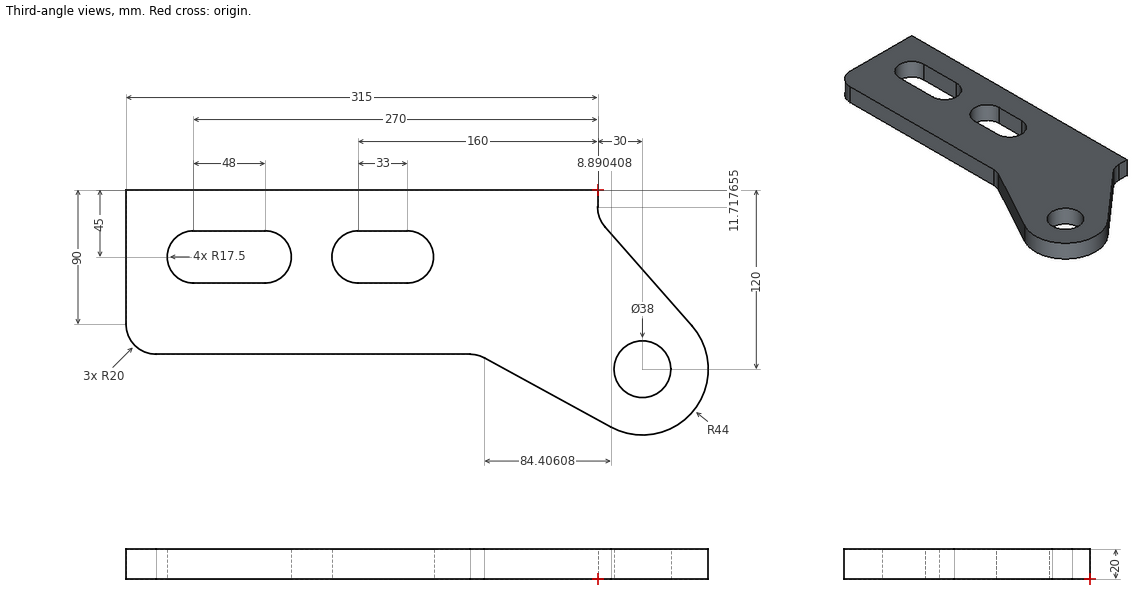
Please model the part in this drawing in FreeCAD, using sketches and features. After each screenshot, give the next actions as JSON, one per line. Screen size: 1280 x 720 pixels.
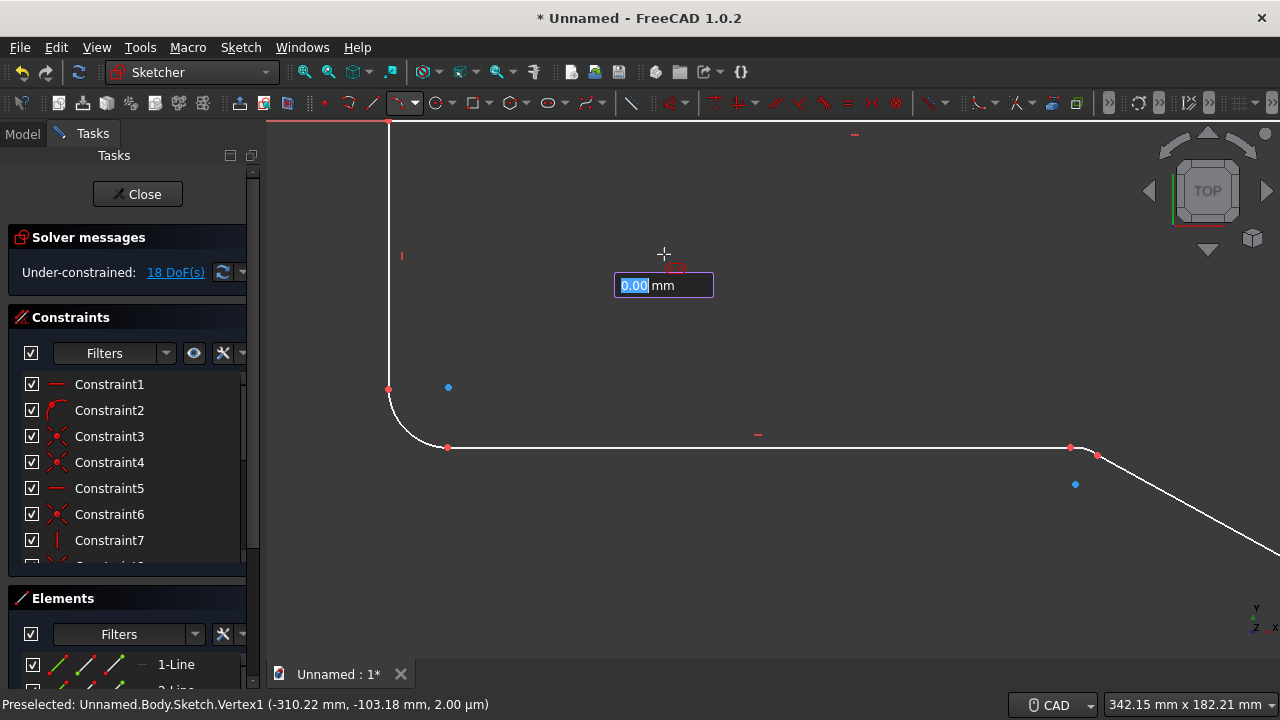
{"action": "left_click", "coordinate": [593, 202]}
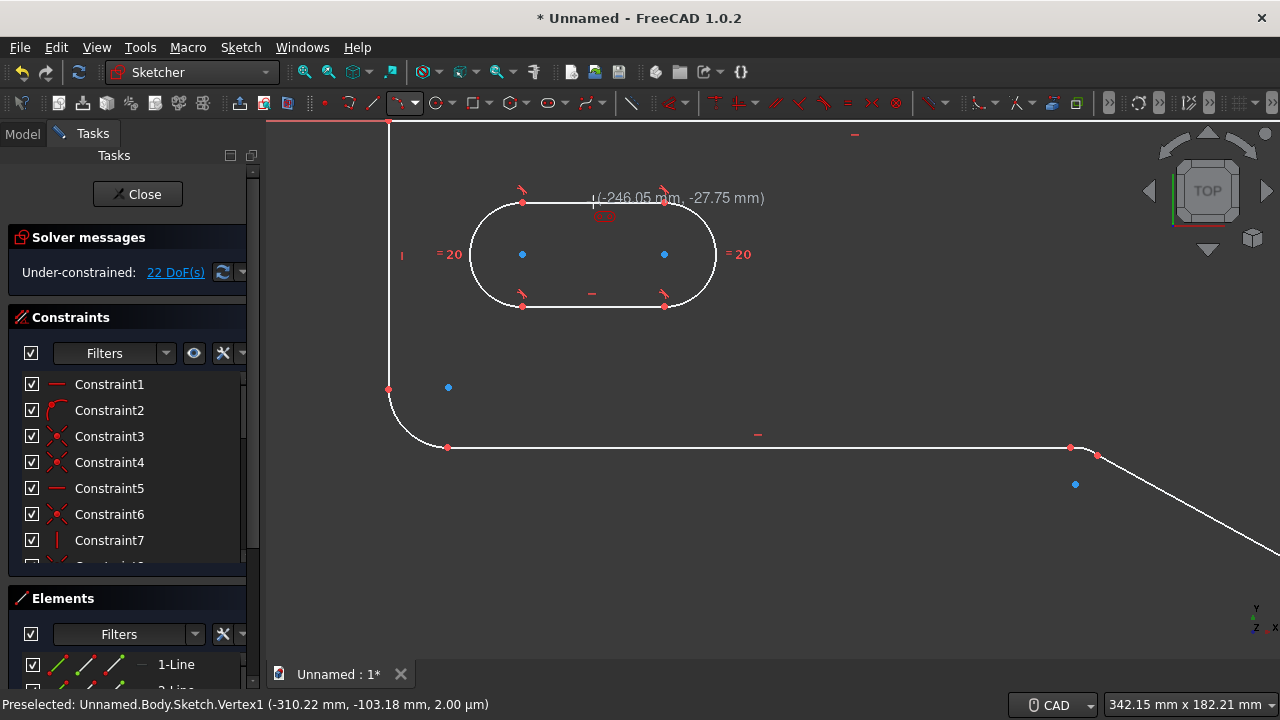
{"action": "left_click", "coordinate": [848, 254]}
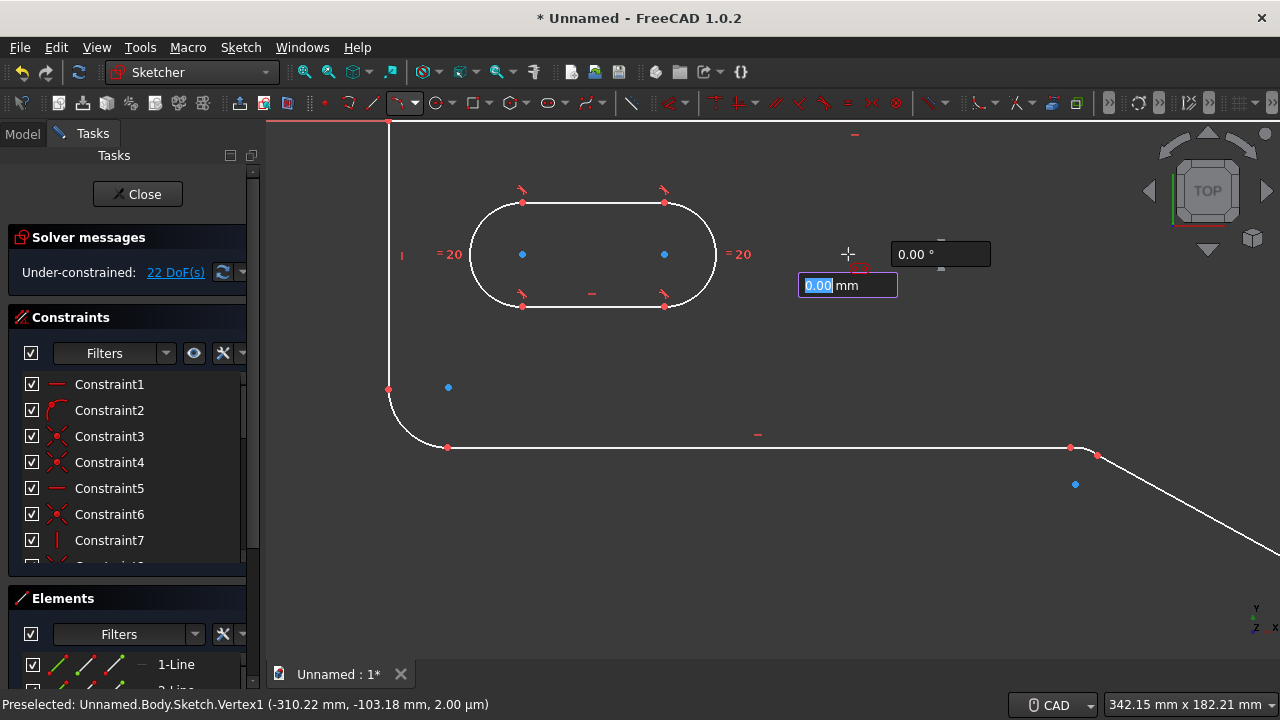
{"action": "left_click", "coordinate": [946, 254]}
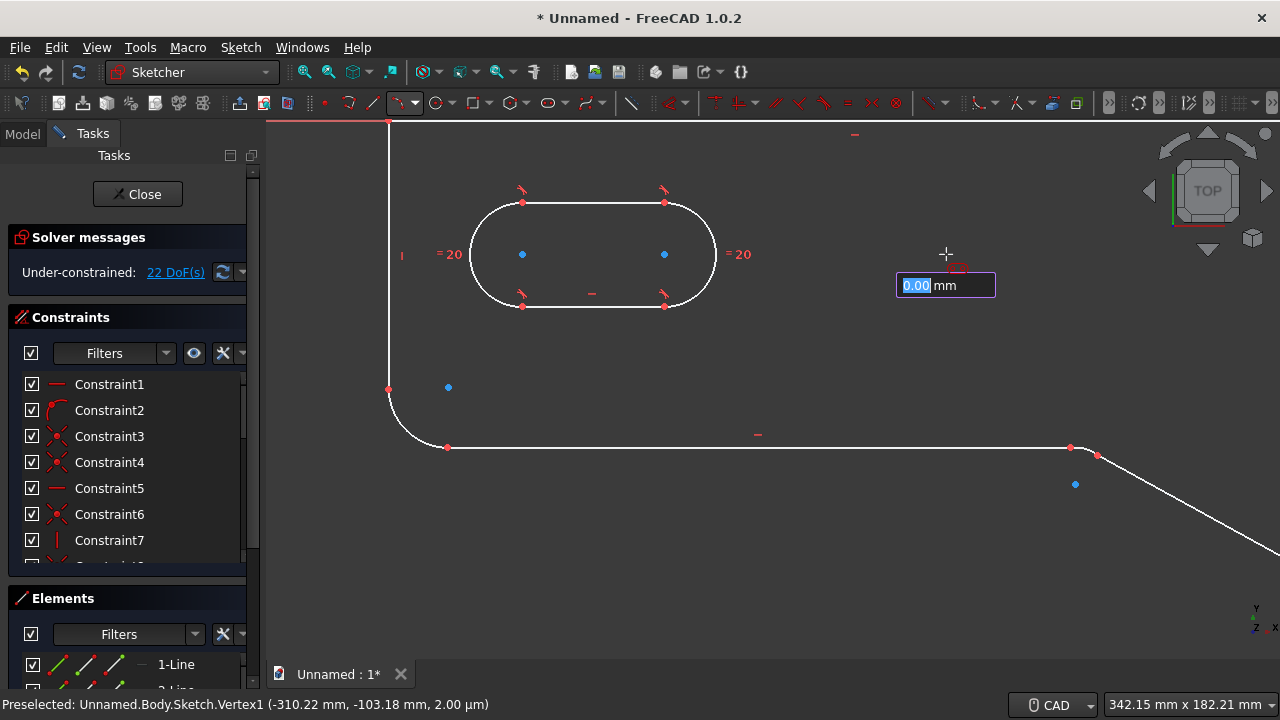
{"action": "left_click", "coordinate": [897, 202]}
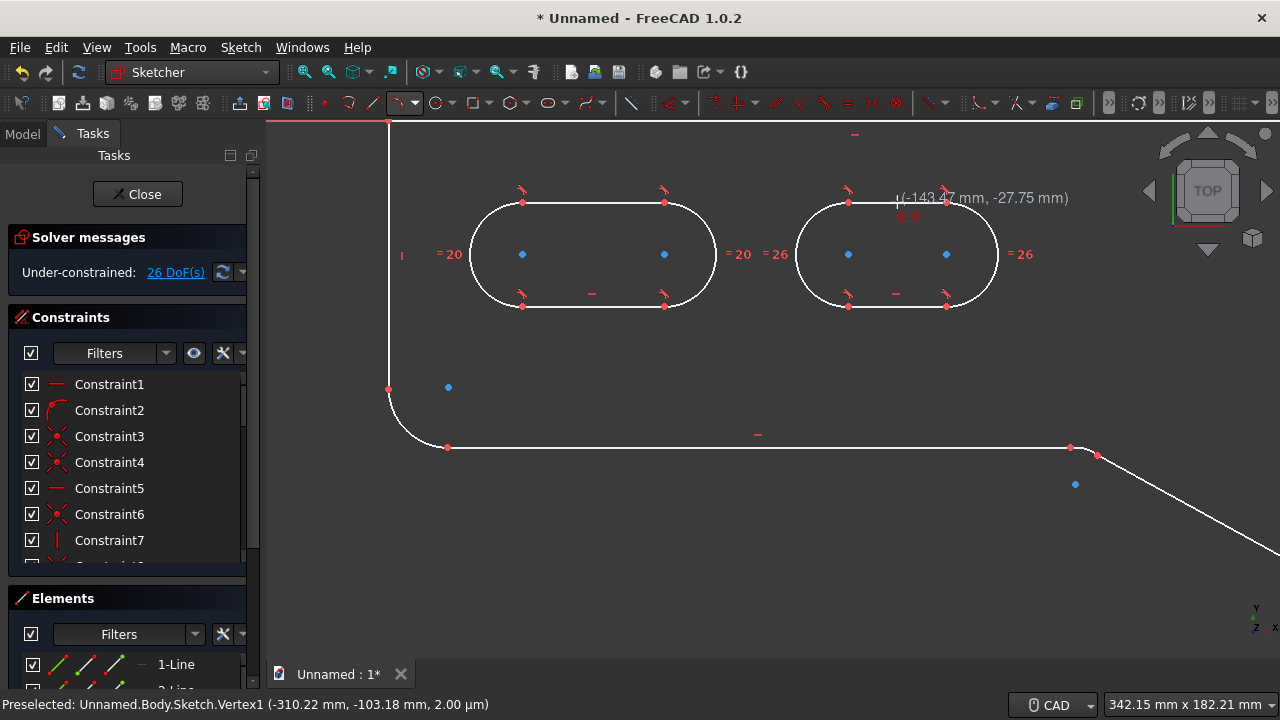
{"action": "left_click", "coordinate": [436, 104]}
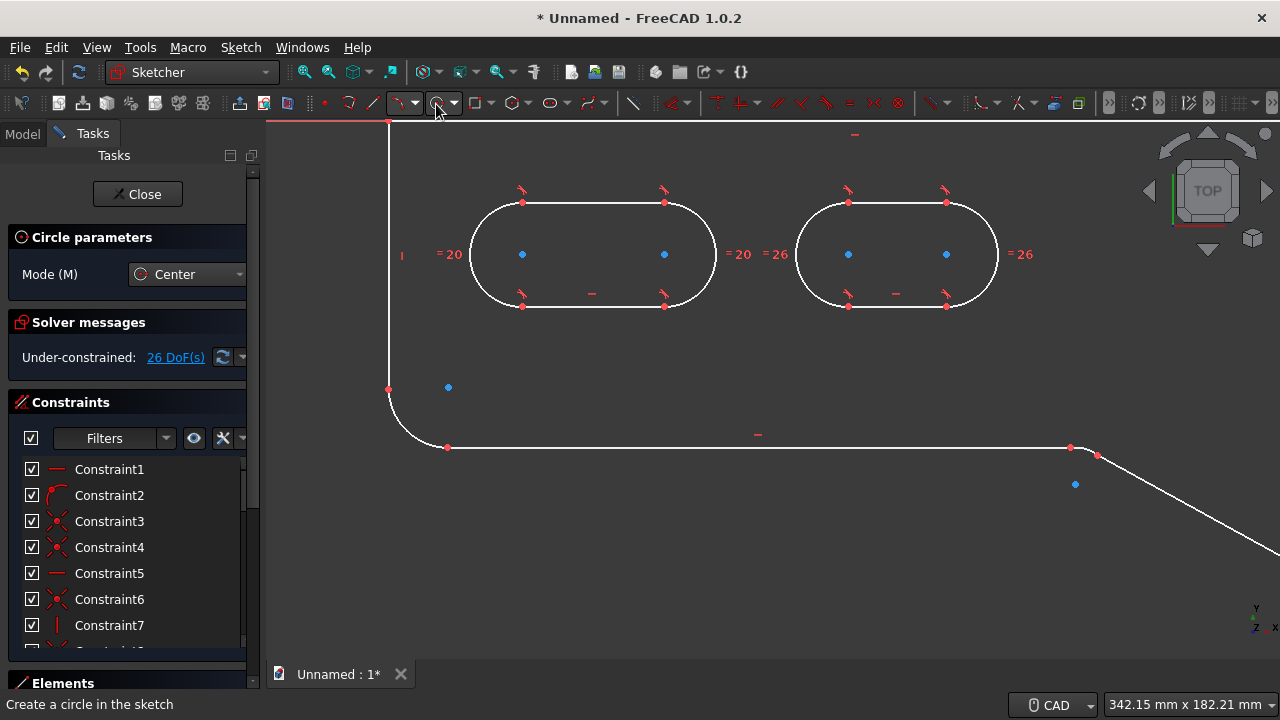
{"action": "scroll", "coordinate": [405, 429], "scroll_direction": "down", "scroll_amount": 3}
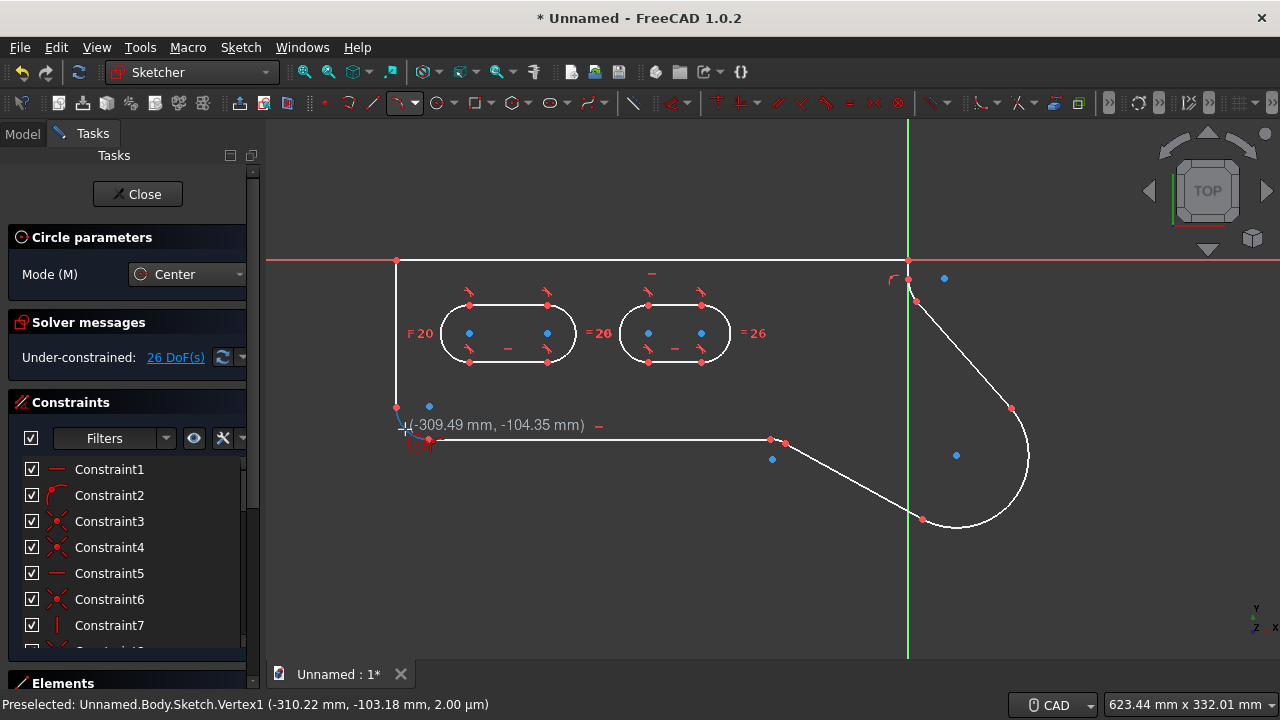
{"action": "left_click", "coordinate": [957, 455]}
{"action": "mouse_move", "coordinate": [979, 433]}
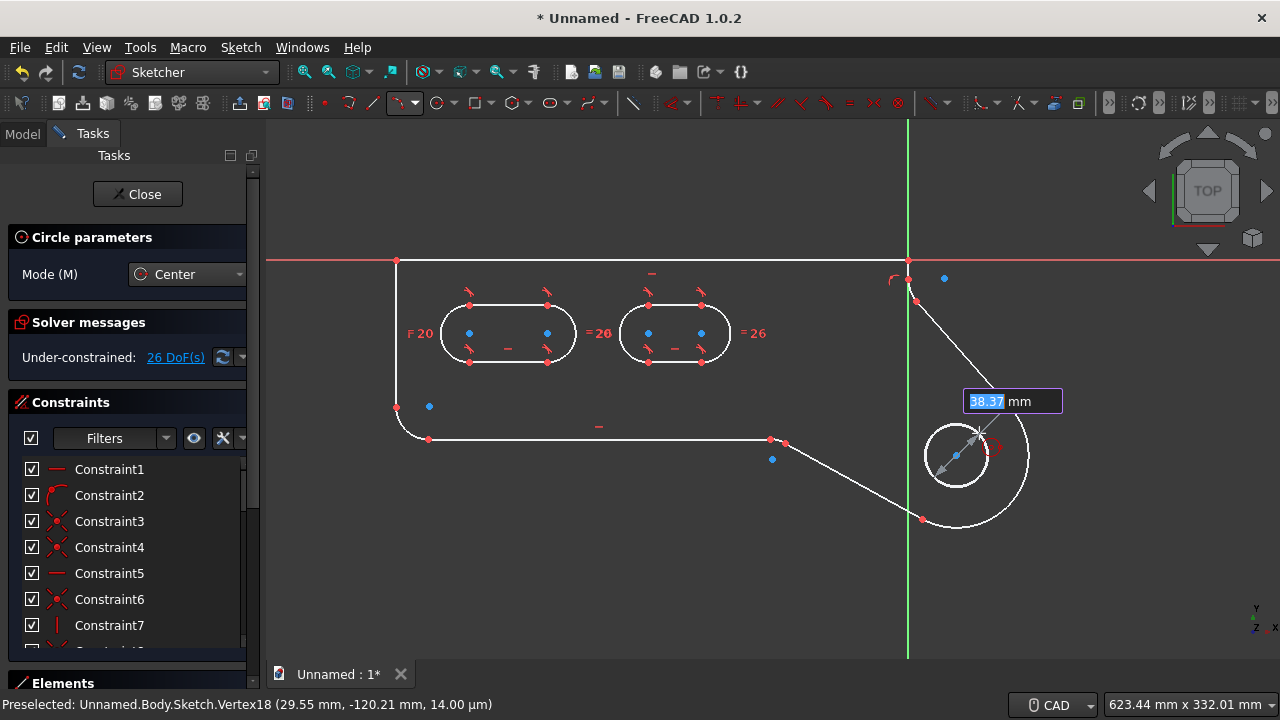
{"action": "type", "text": "38"}
{"action": "key", "text": "Return"}
{"action": "key", "text": "Escape"}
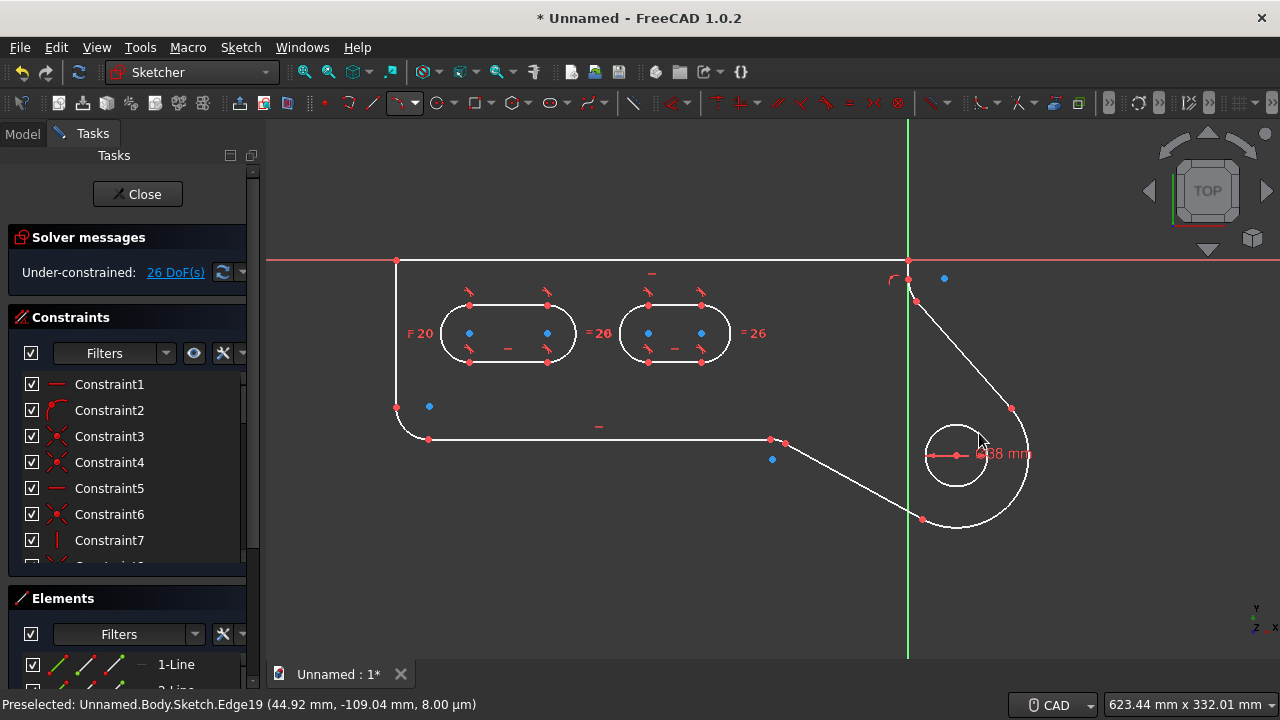
{"action": "left_click", "coordinate": [531, 440]}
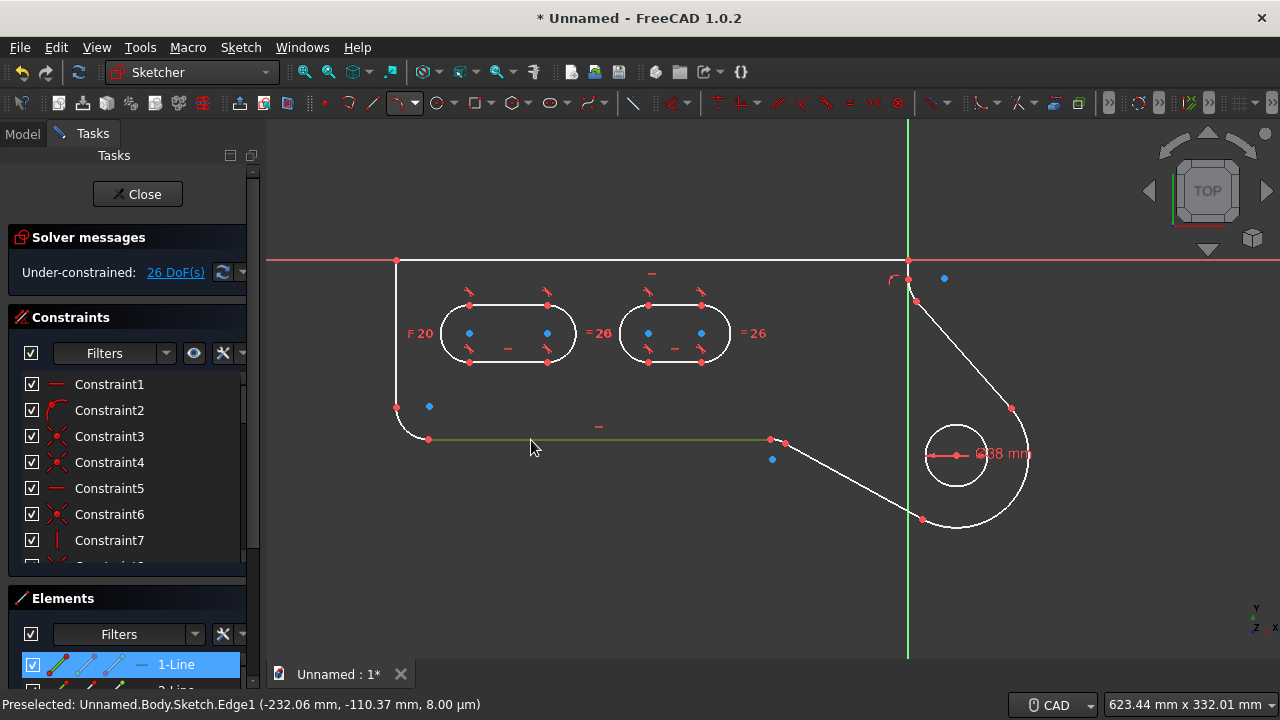
{"action": "scroll", "coordinate": [778, 440], "scroll_direction": "up", "scroll_amount": 3}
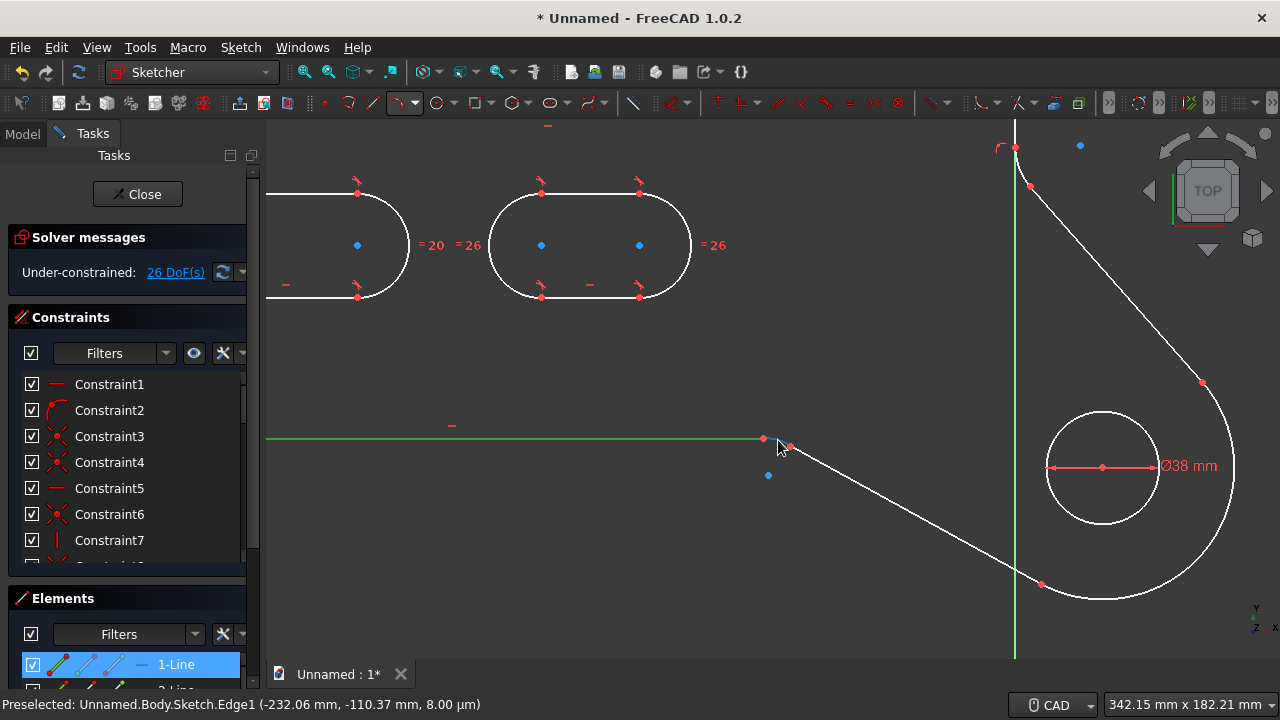
{"action": "left_click", "coordinate": [778, 440]}